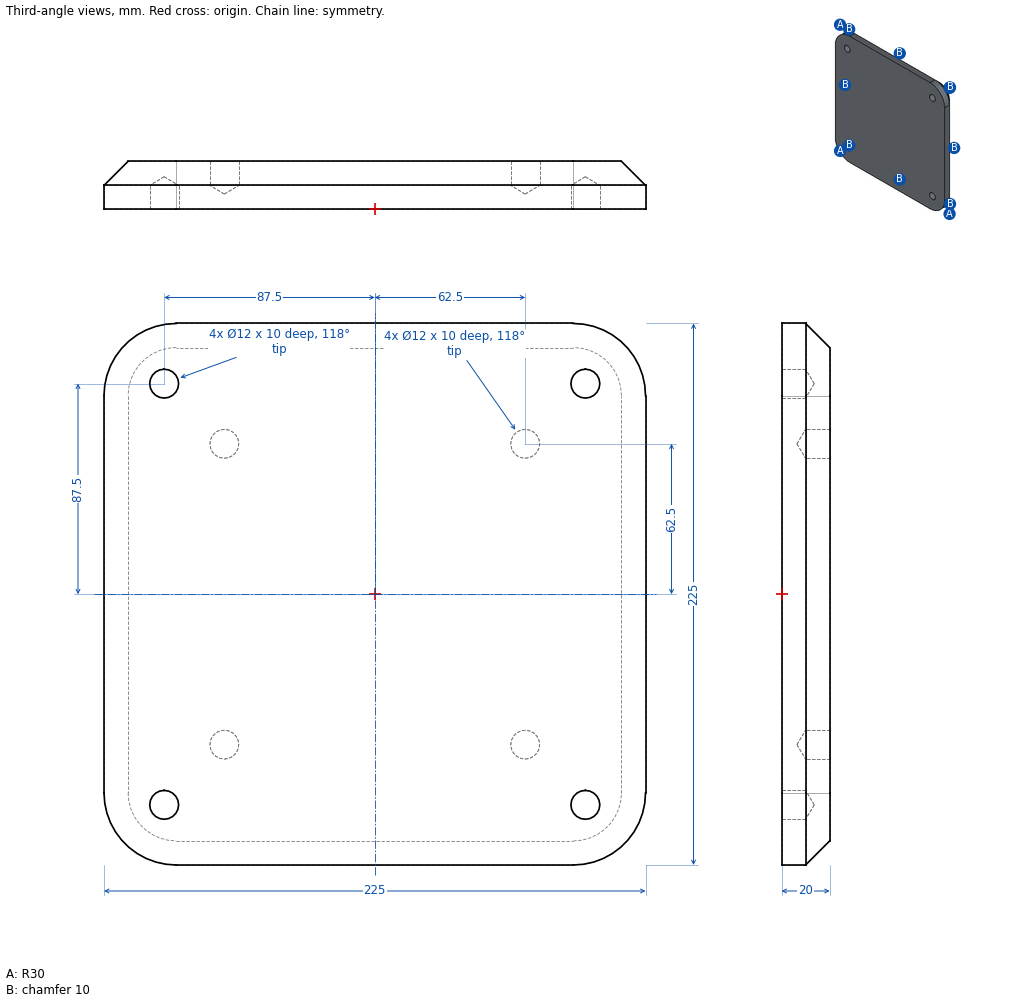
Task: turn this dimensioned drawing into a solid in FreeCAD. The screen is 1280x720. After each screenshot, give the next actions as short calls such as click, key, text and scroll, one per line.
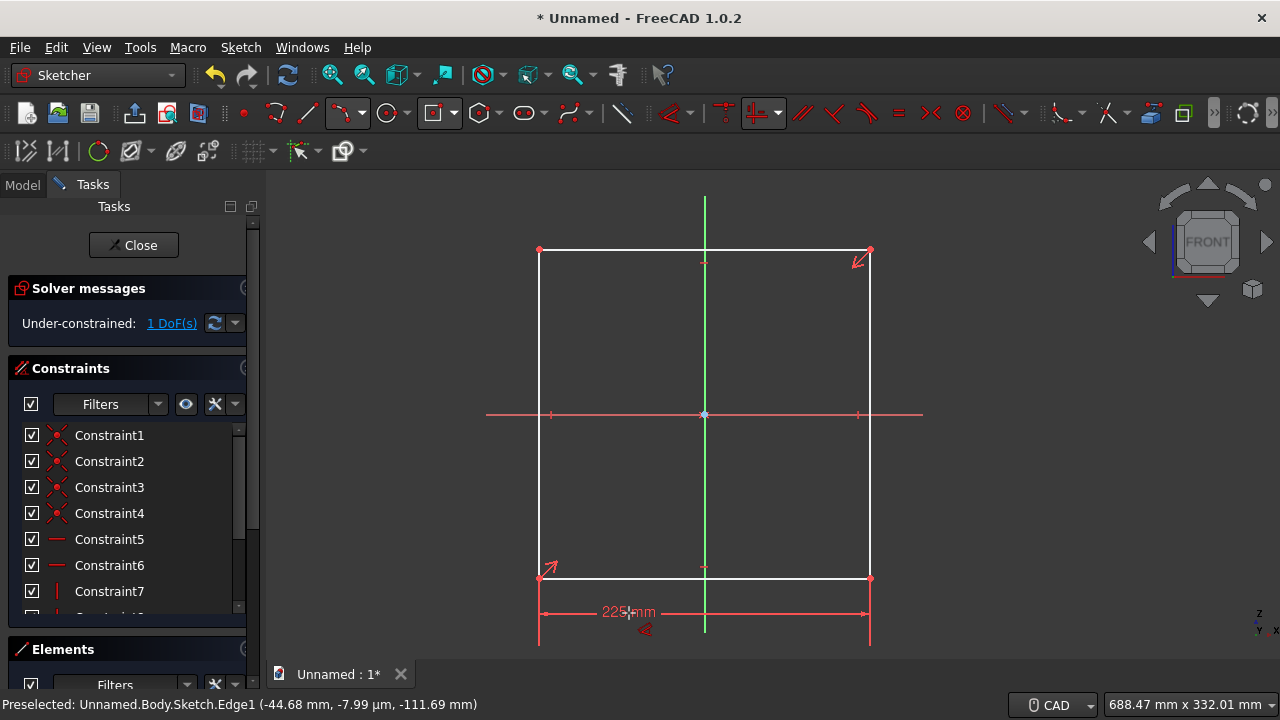
click(870, 480)
click(904, 339)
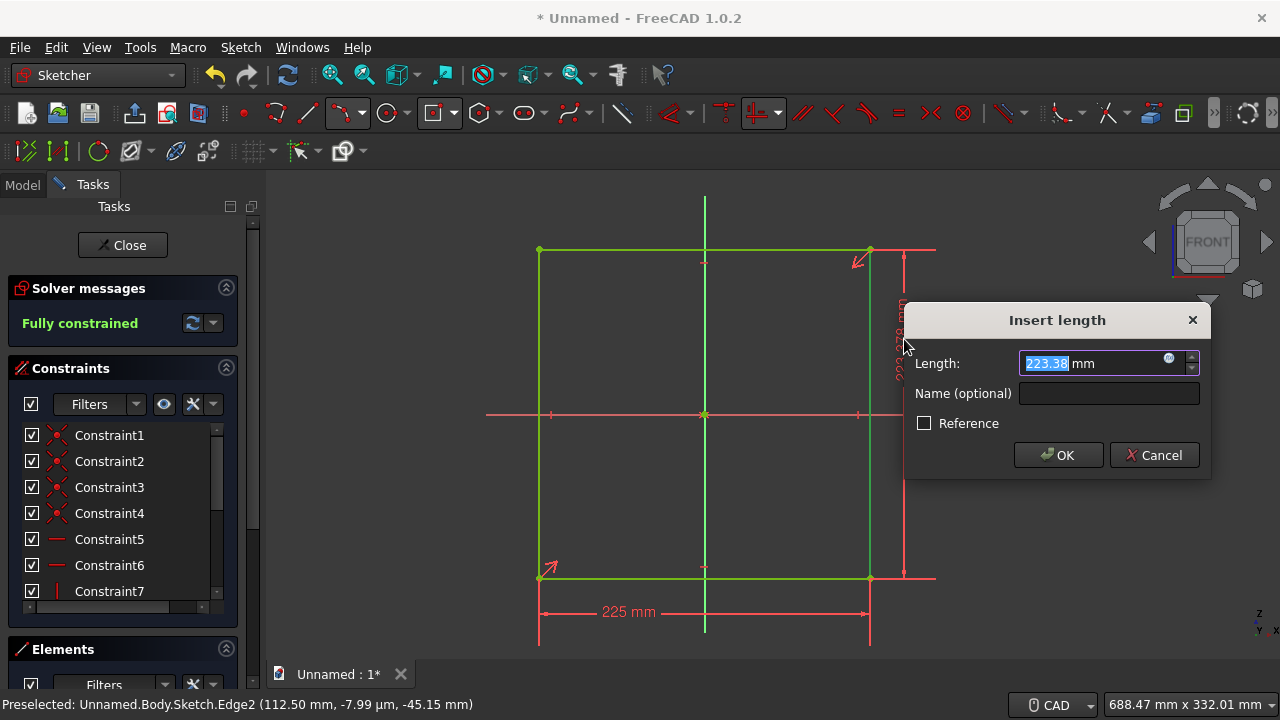
text(225)
key(Return)
key(Escape)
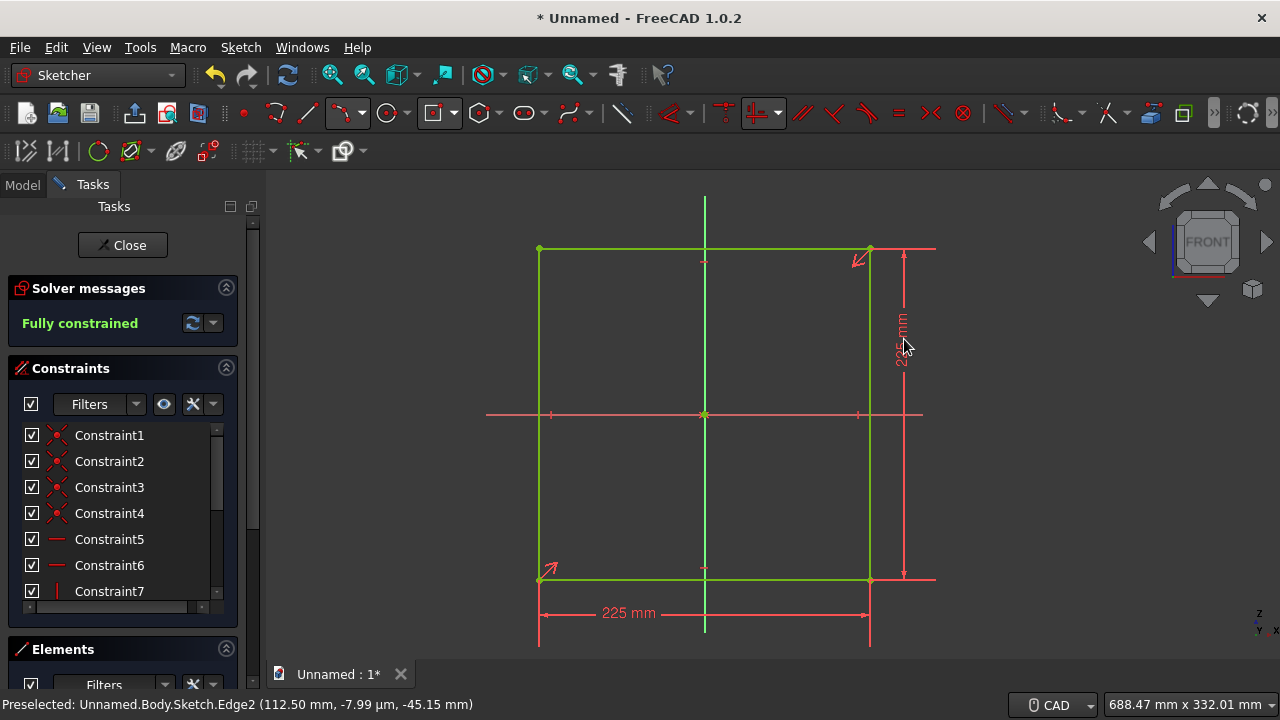
click(123, 245)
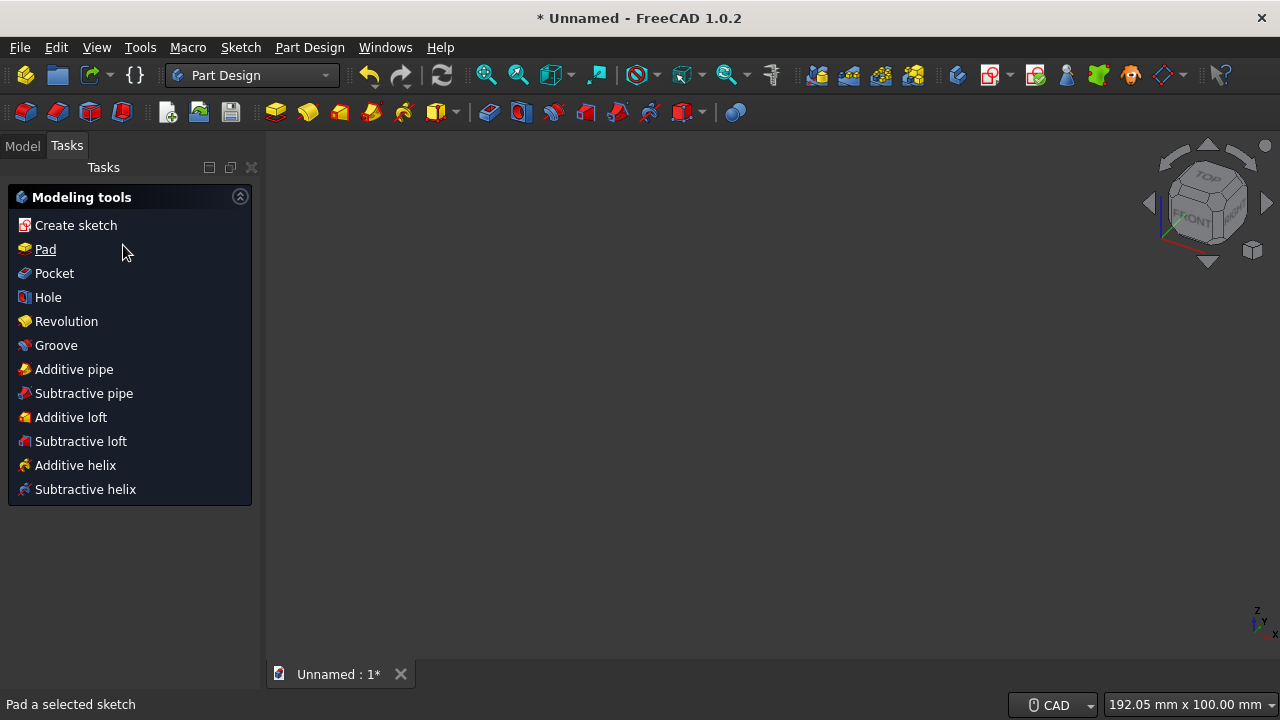
click(276, 112)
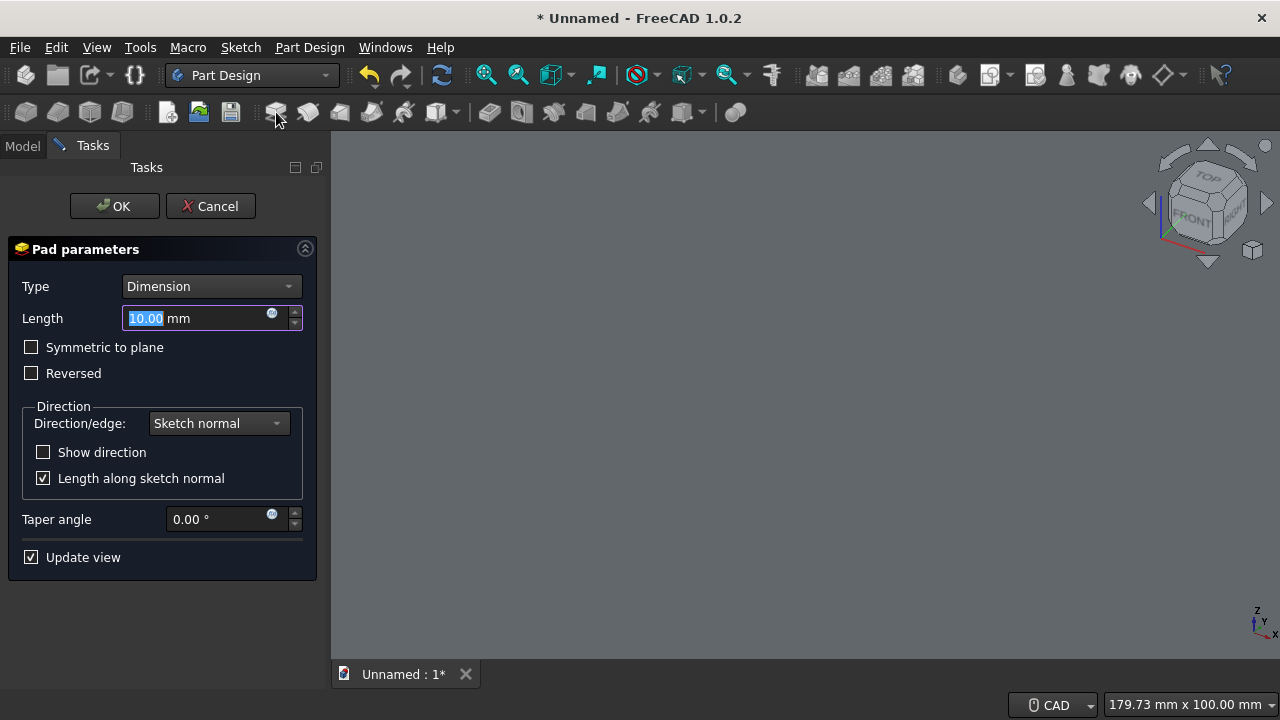
text(20)
key(Tab)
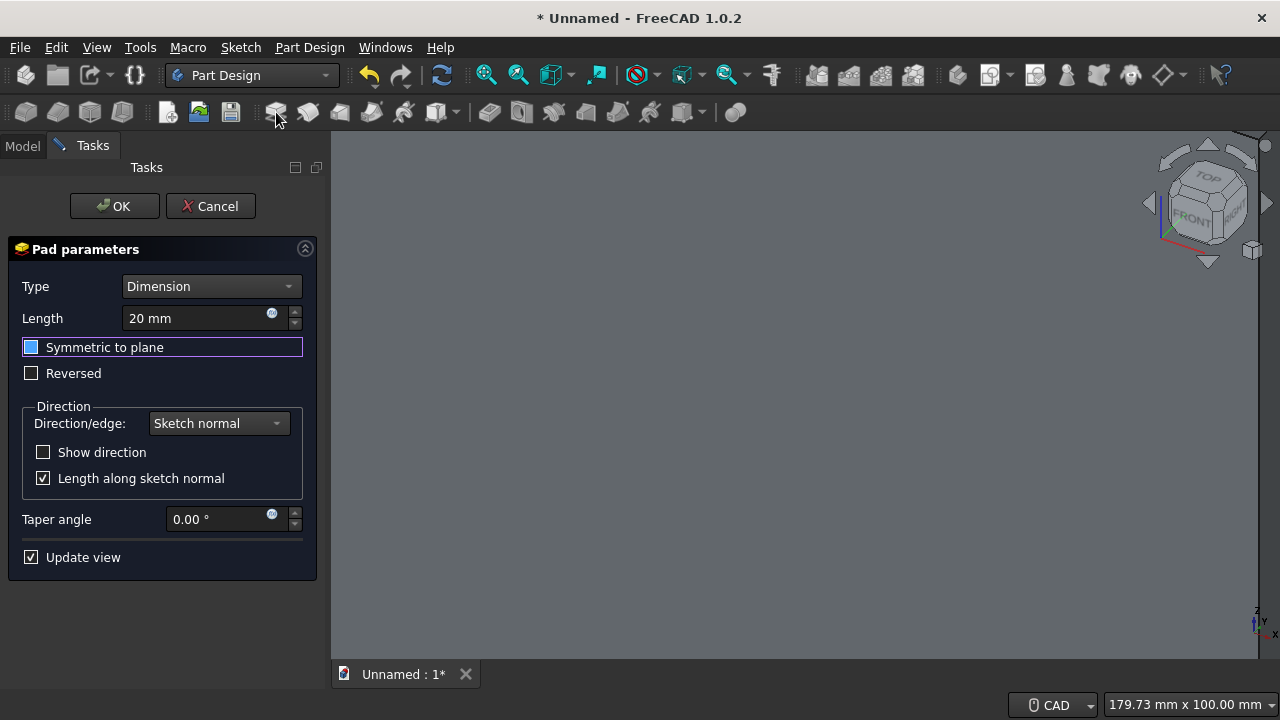
click(30, 373)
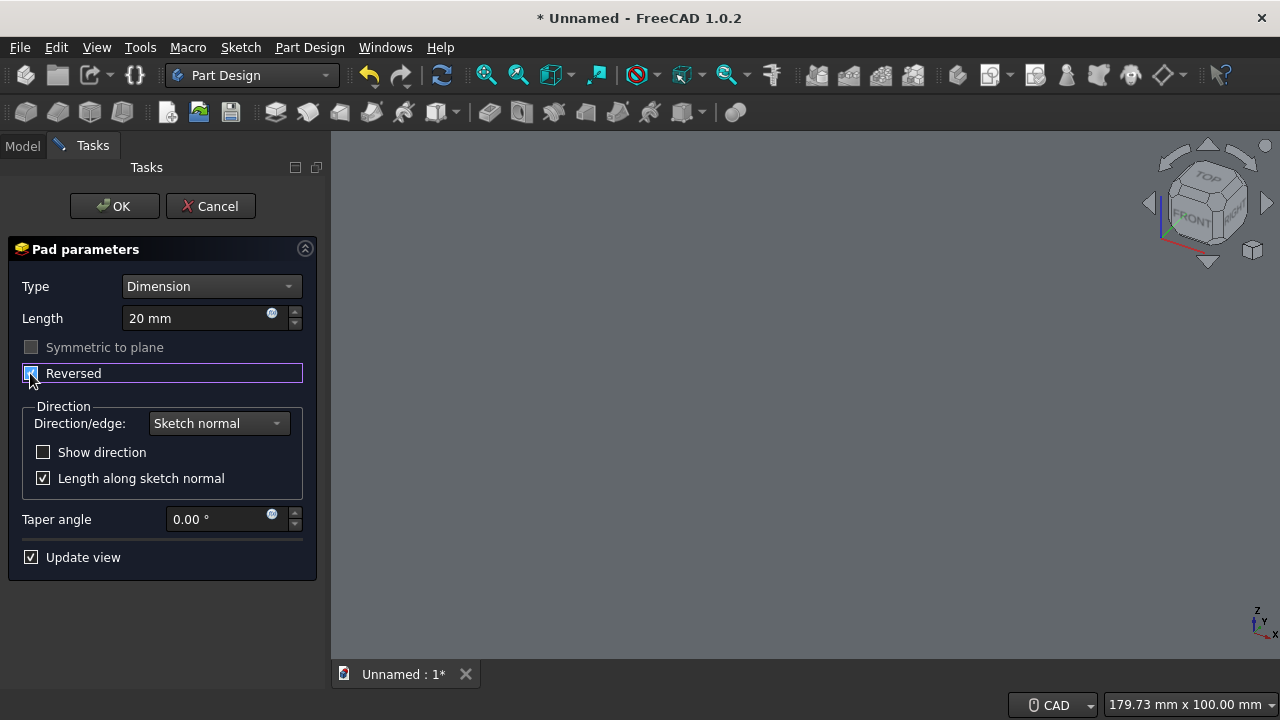
click(115, 206)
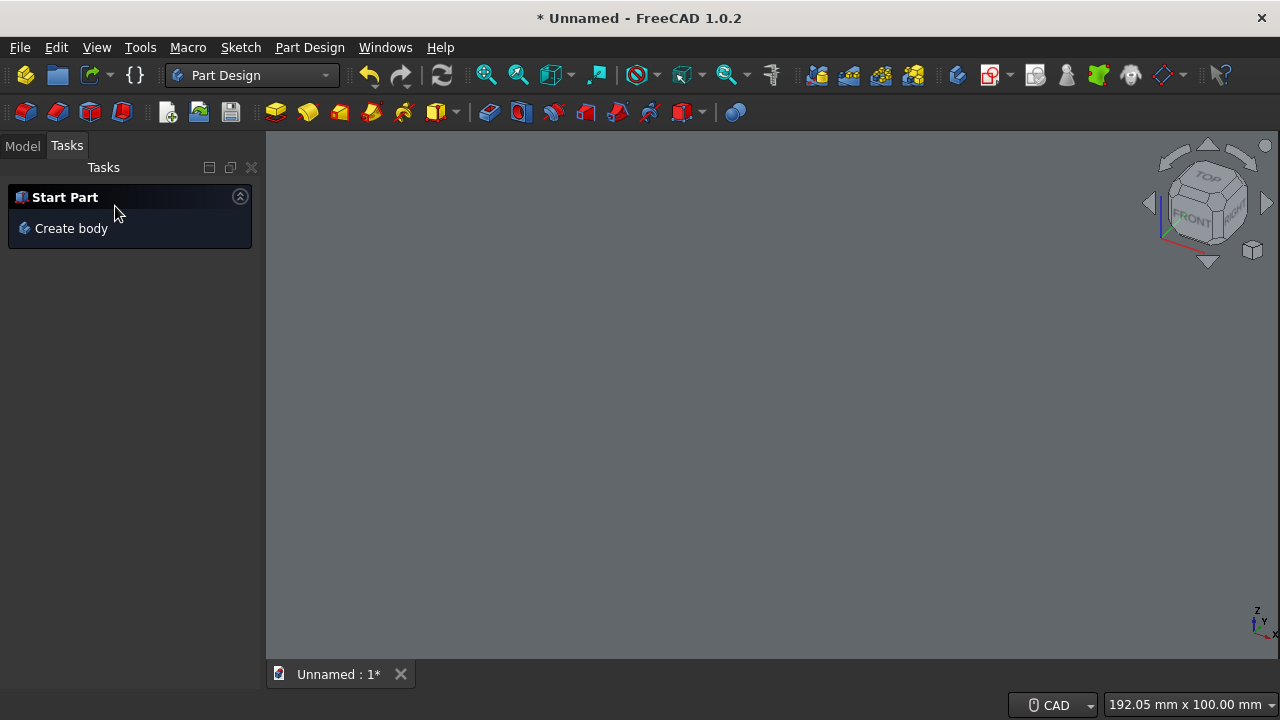
click(488, 76)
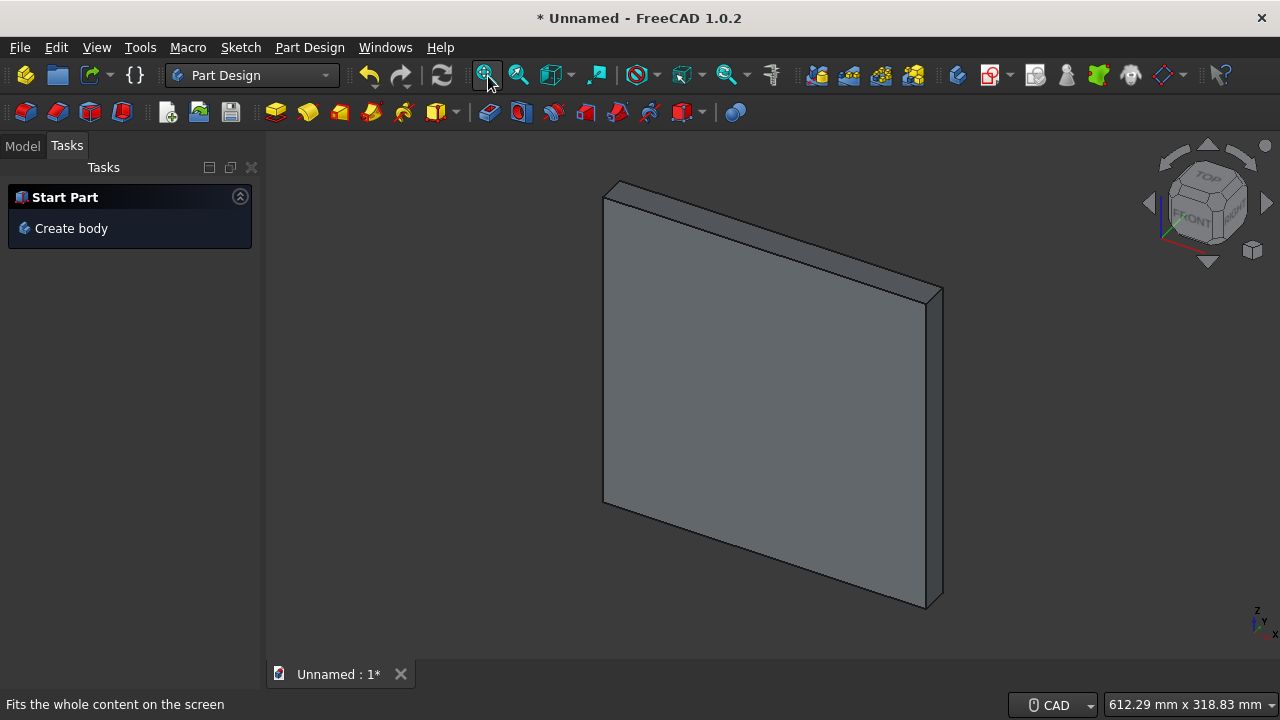
click(934, 295)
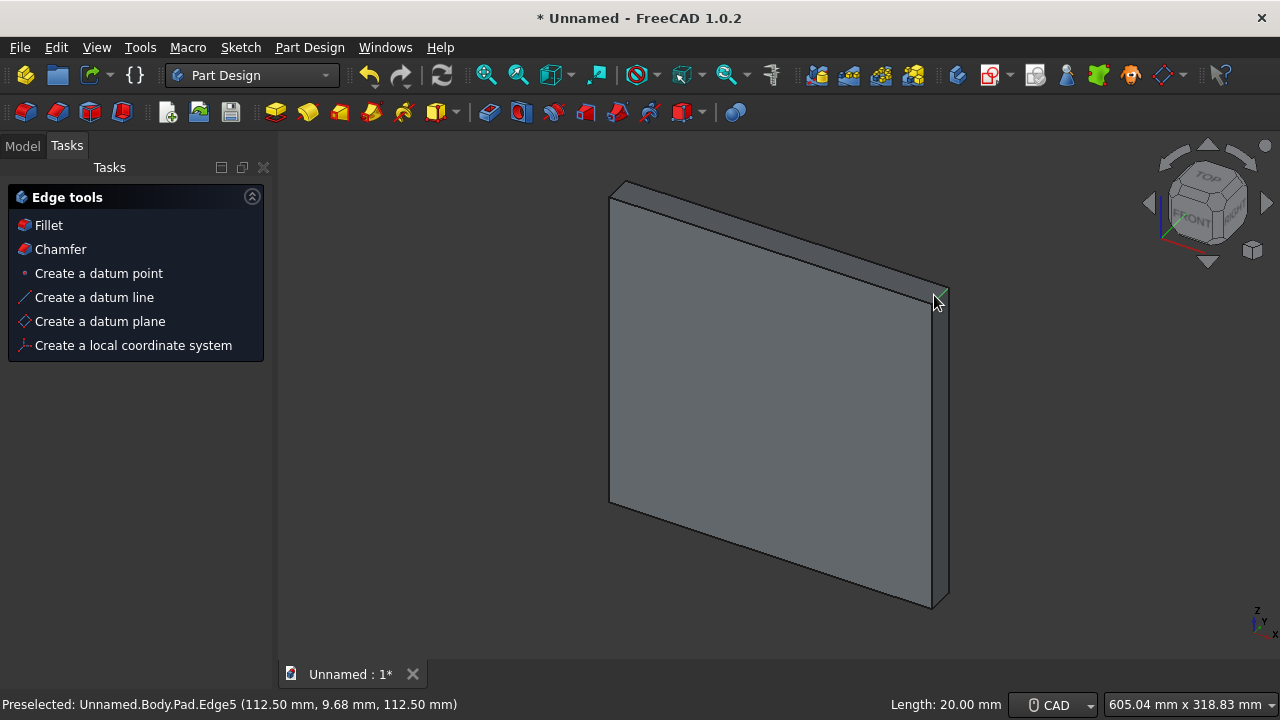
key(0)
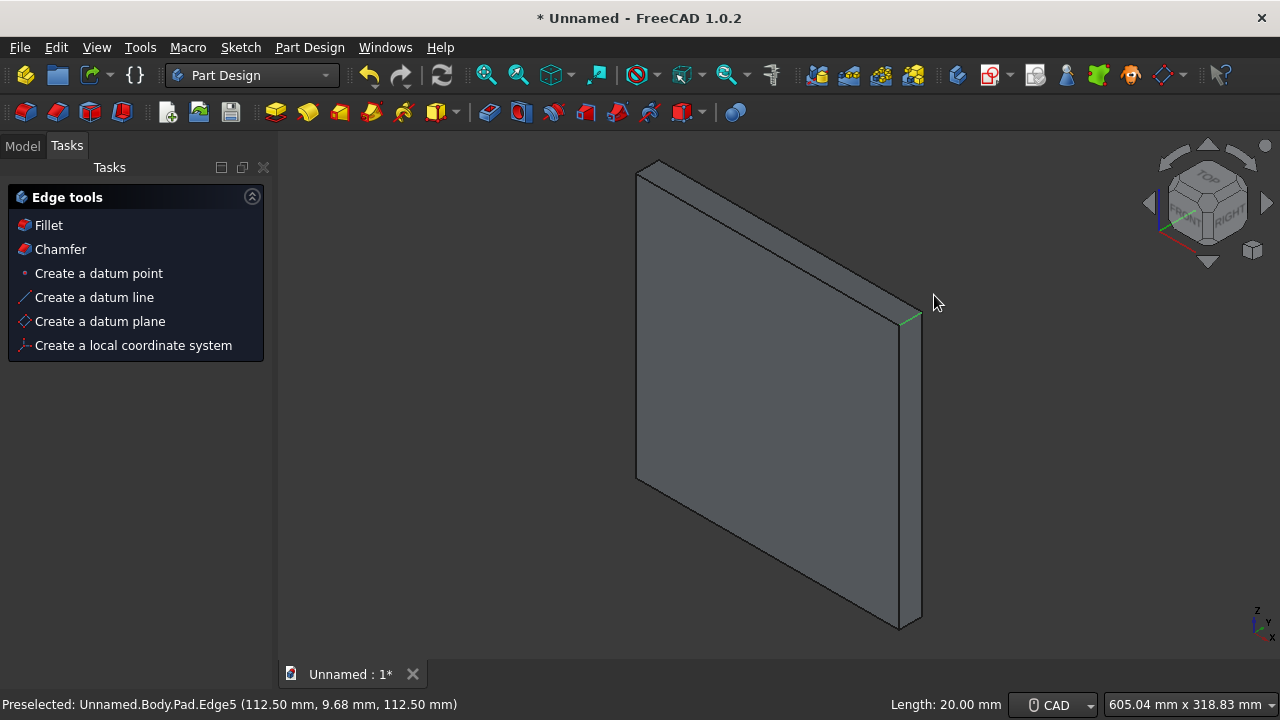
key(2)